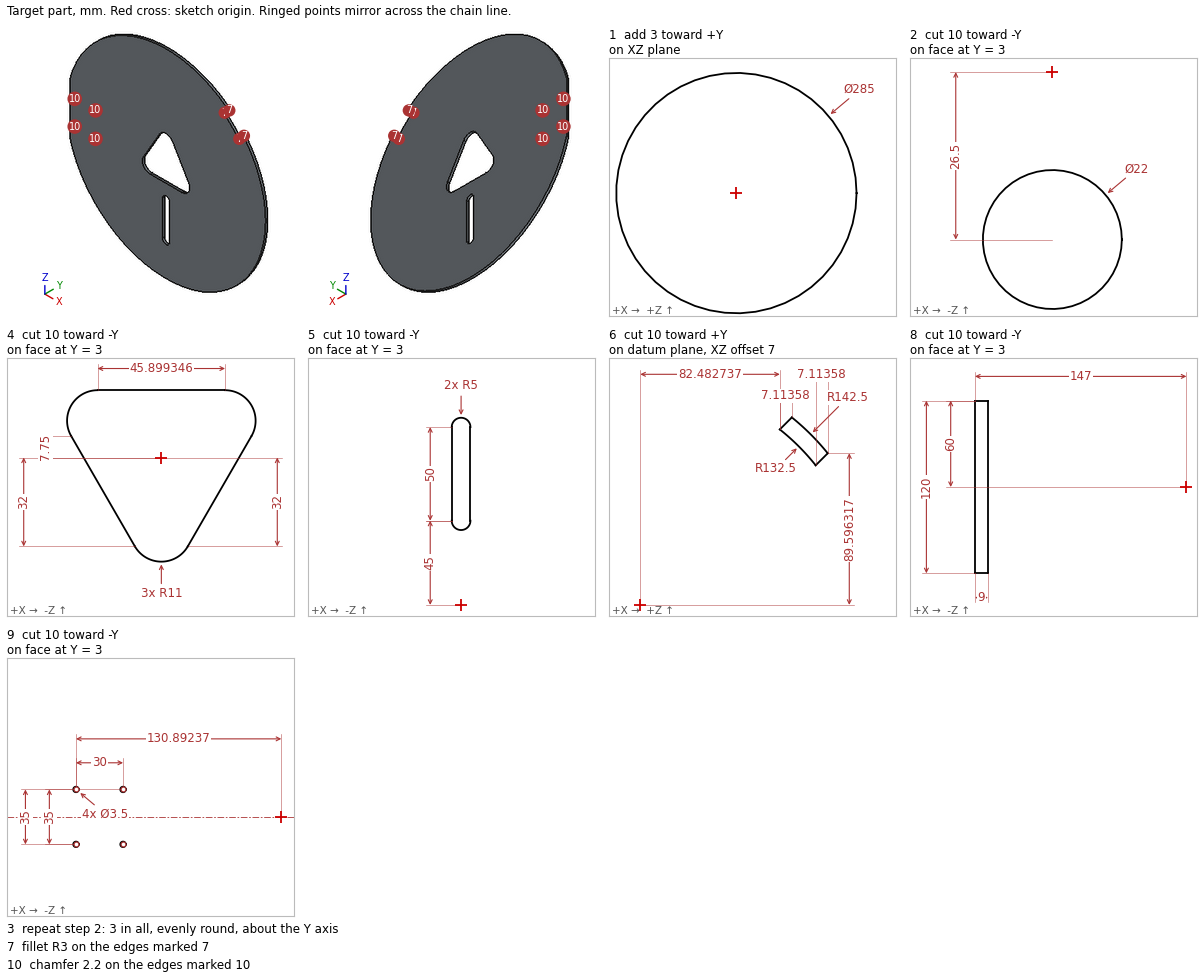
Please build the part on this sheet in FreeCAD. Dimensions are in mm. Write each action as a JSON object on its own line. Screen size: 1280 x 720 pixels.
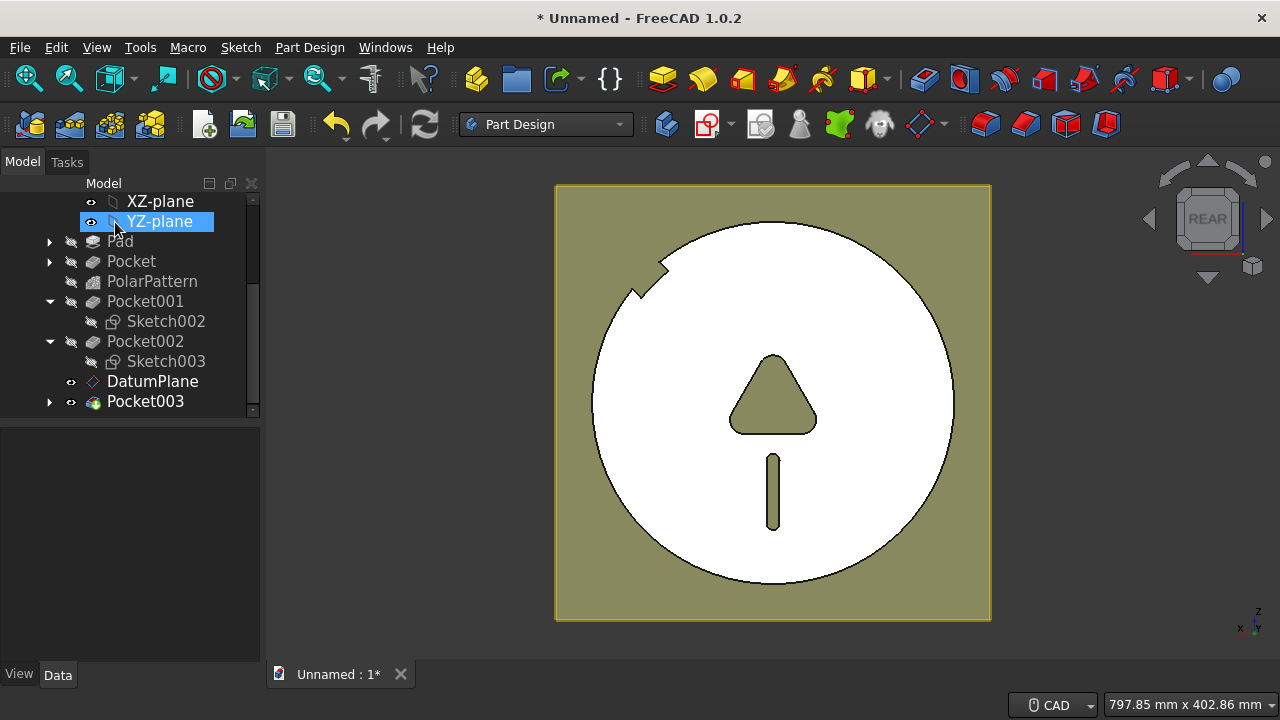
{"action": "left_click", "coordinate": [116, 382]}
{"action": "key", "text": "space"}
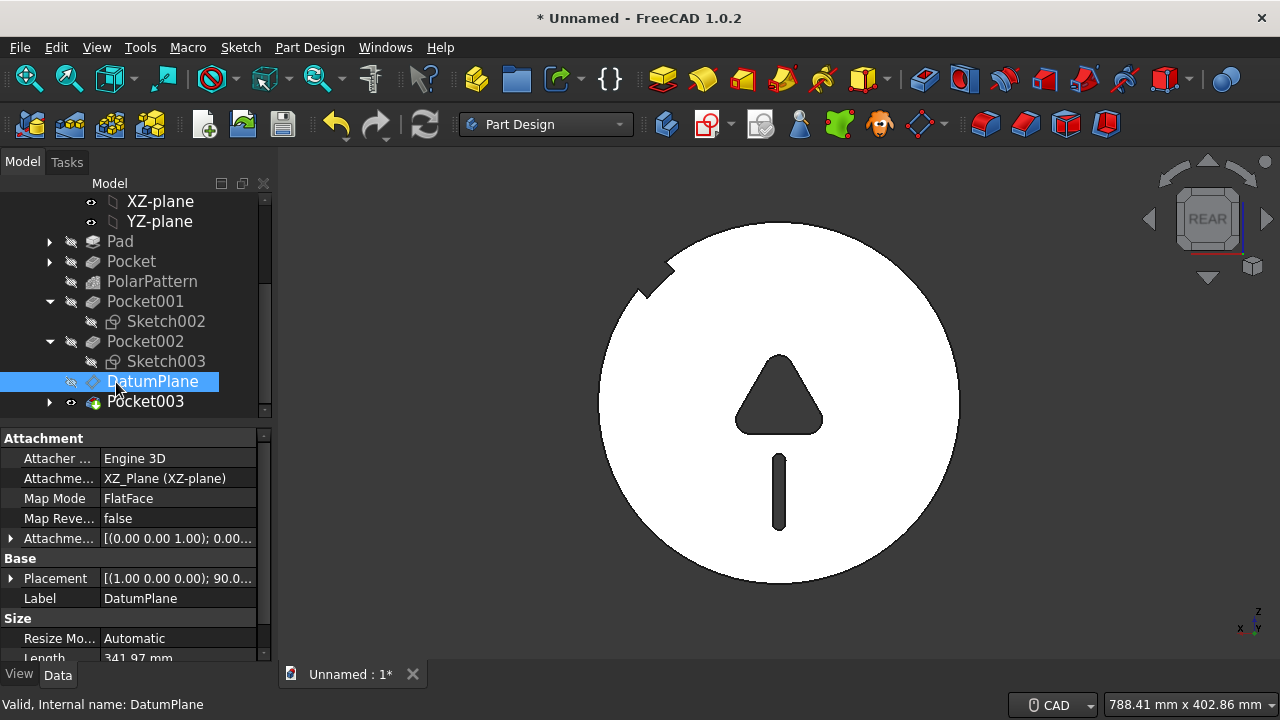
{"action": "scroll", "coordinate": [674, 270], "scroll_direction": "up", "scroll_amount": 12}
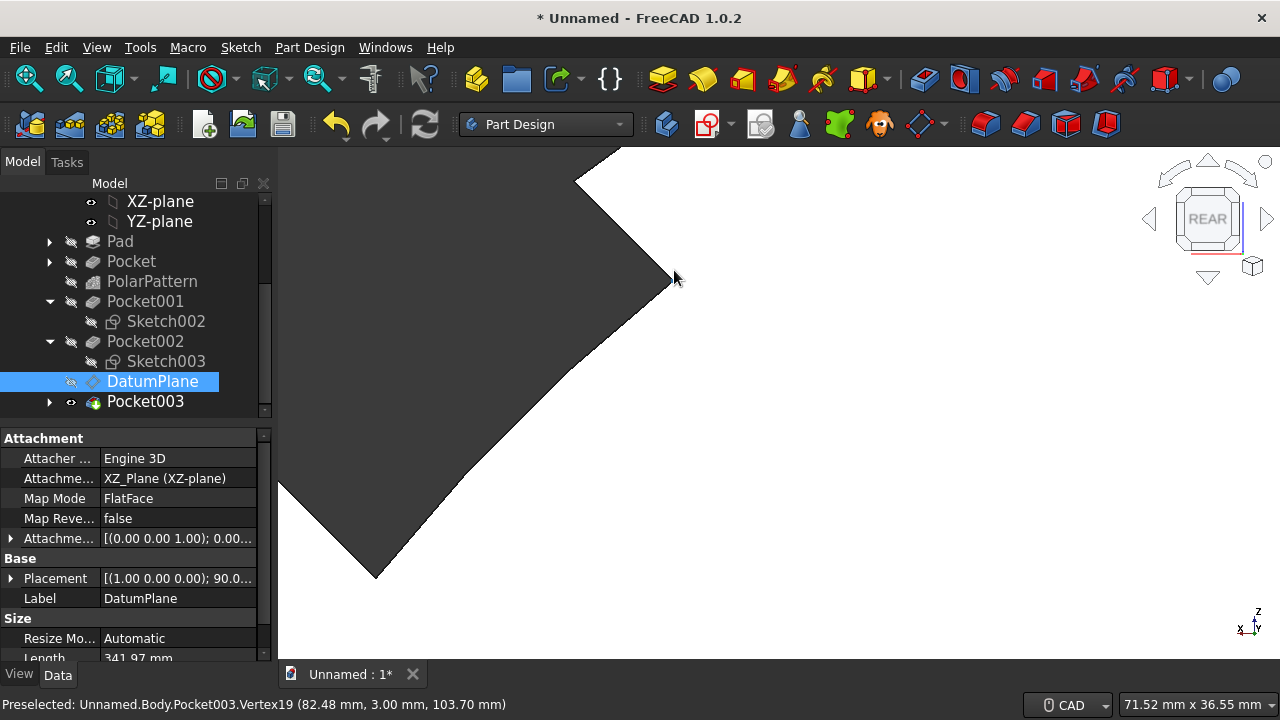
{"action": "key", "text": "v f"}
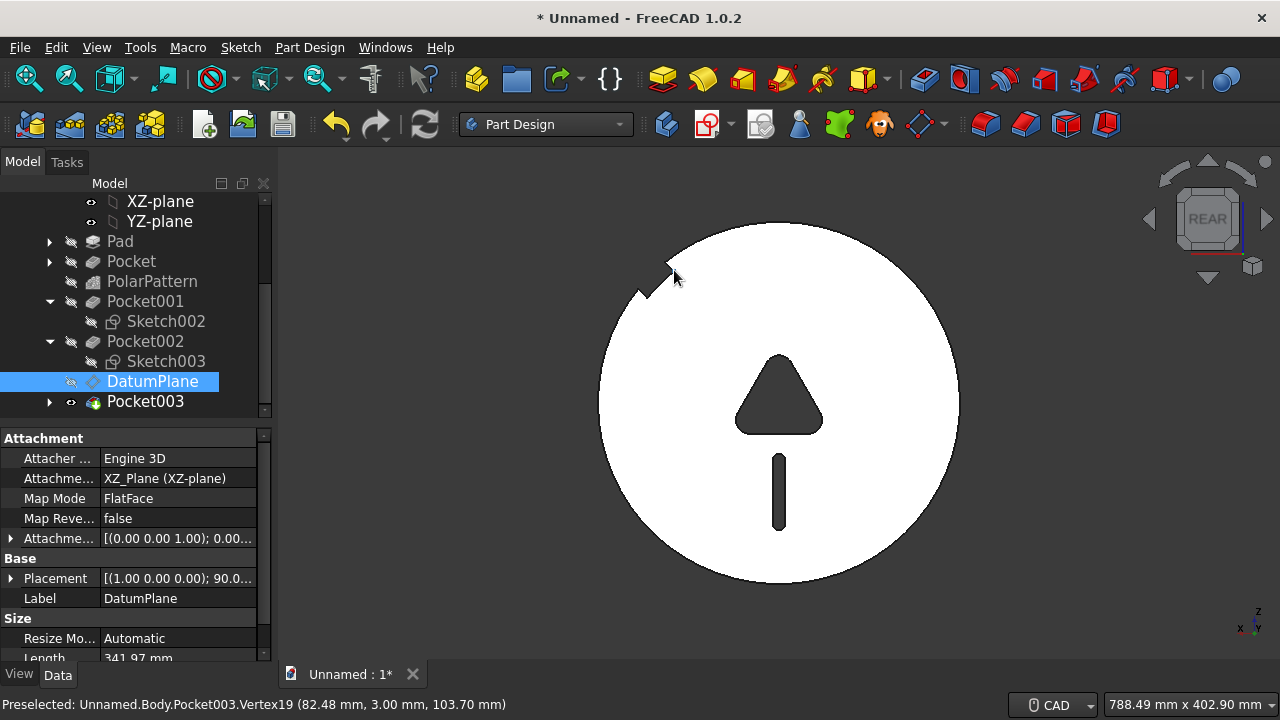
{"action": "key", "text": "0"}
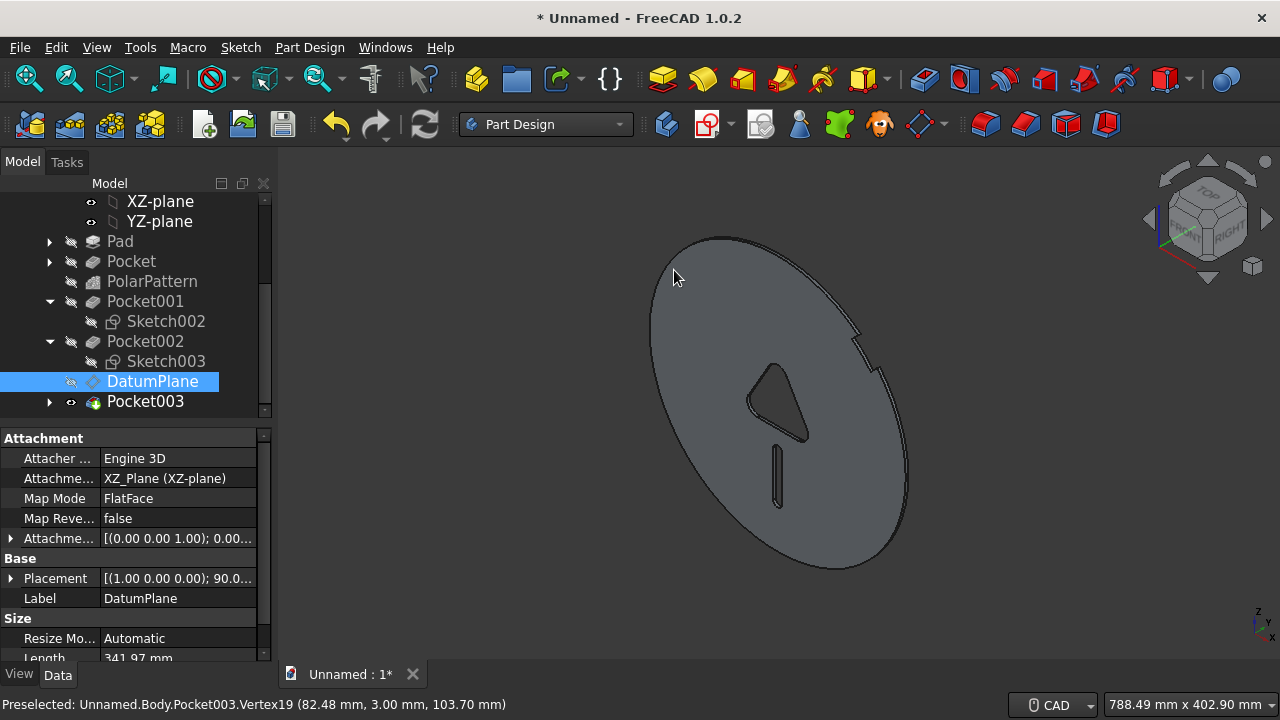
{"action": "scroll", "coordinate": [853, 337], "scroll_direction": "up", "scroll_amount": 12}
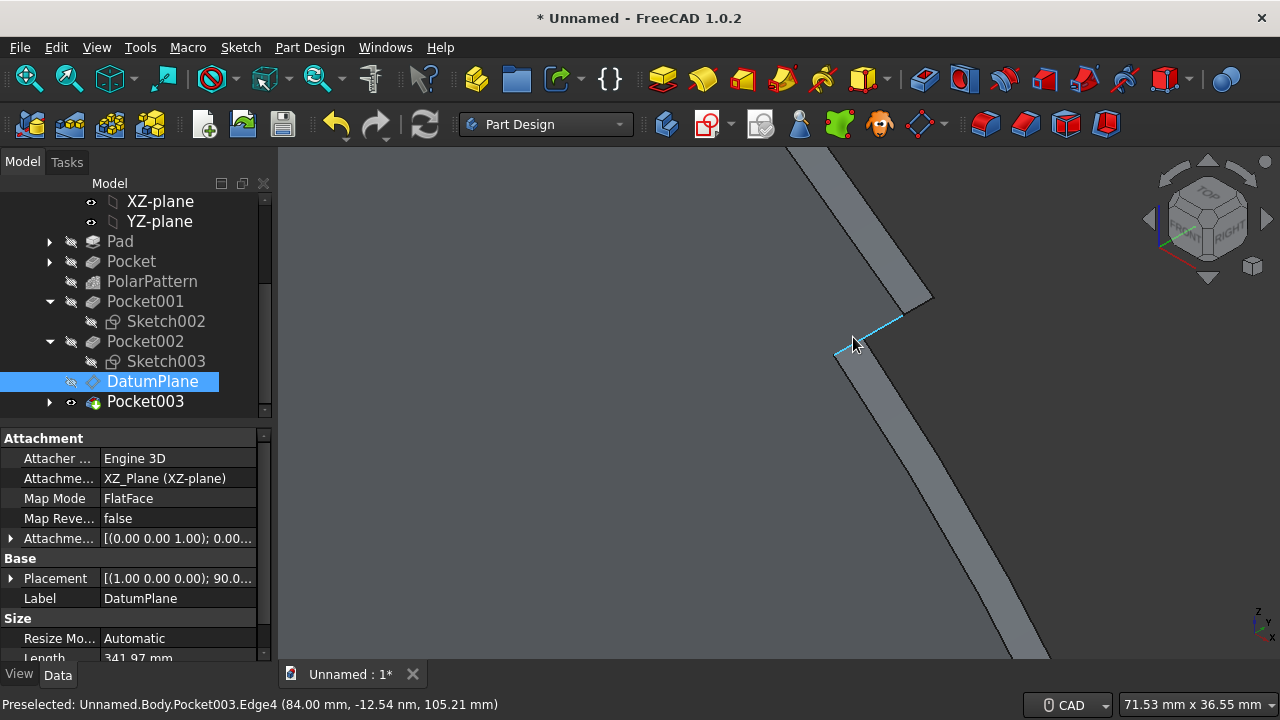
{"action": "left_click", "coordinate": [919, 305]}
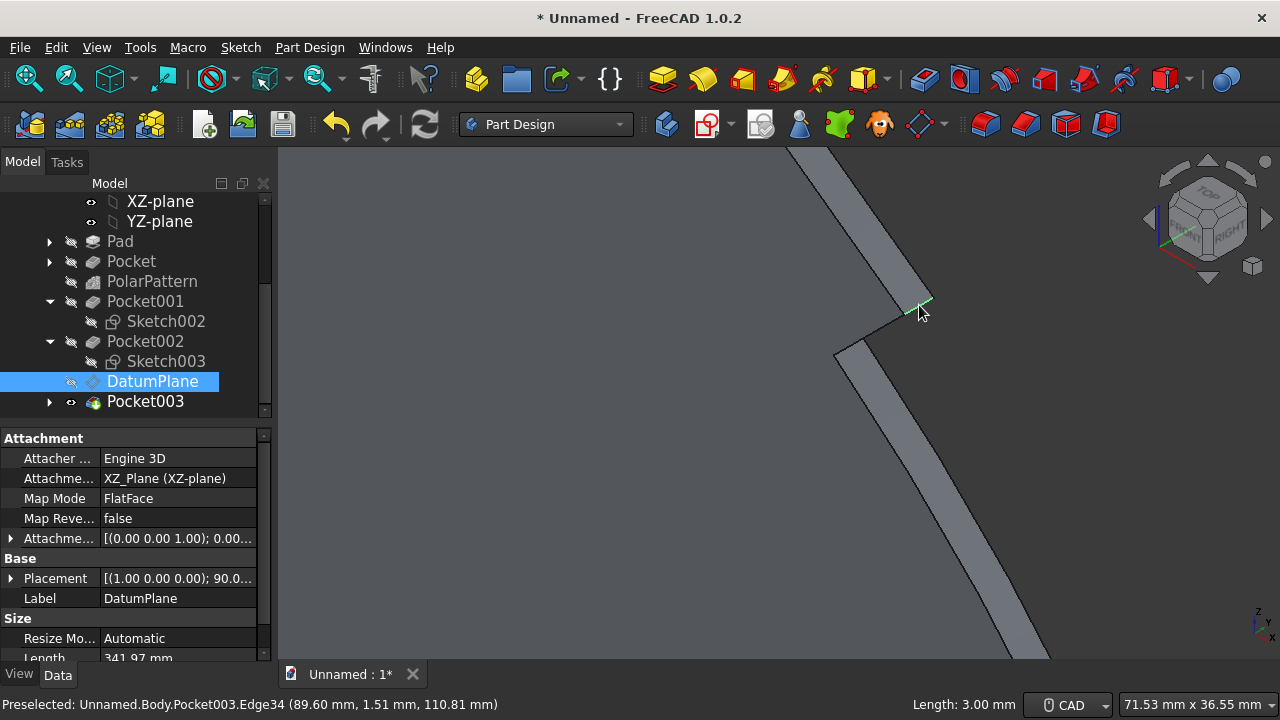
{"action": "left_click", "coordinate": [30, 80]}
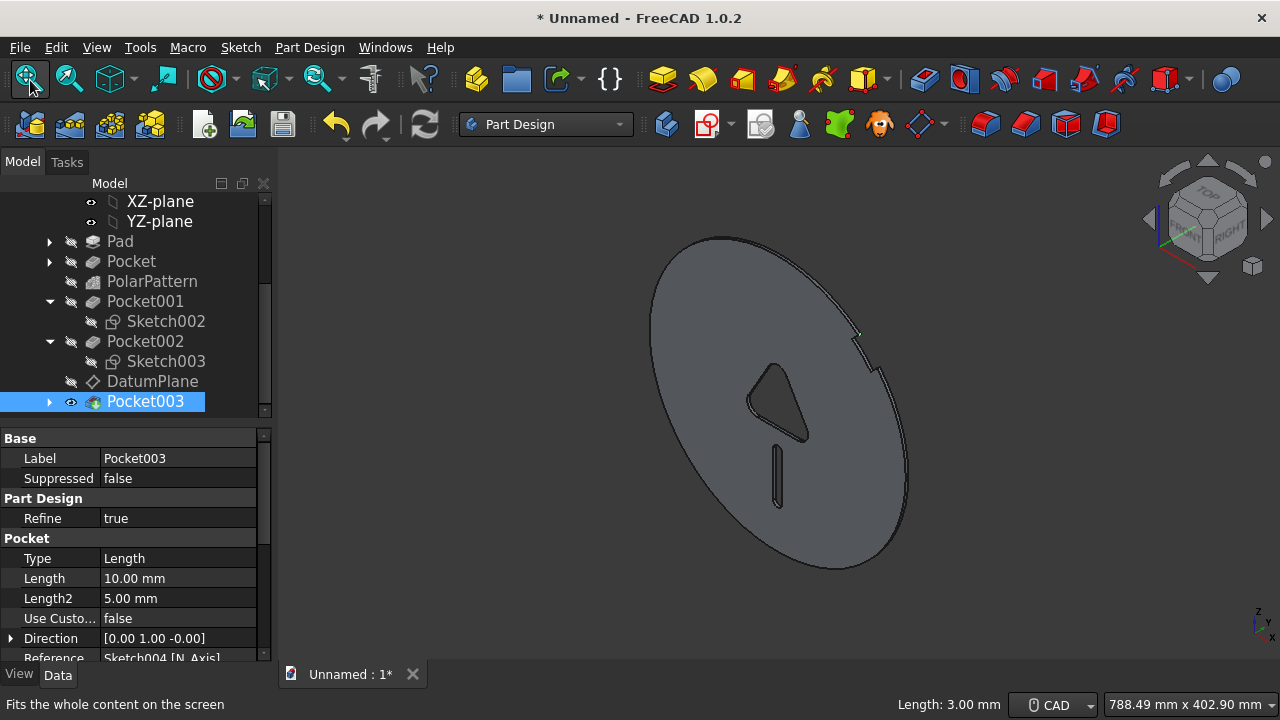
{"action": "key", "text": "2"}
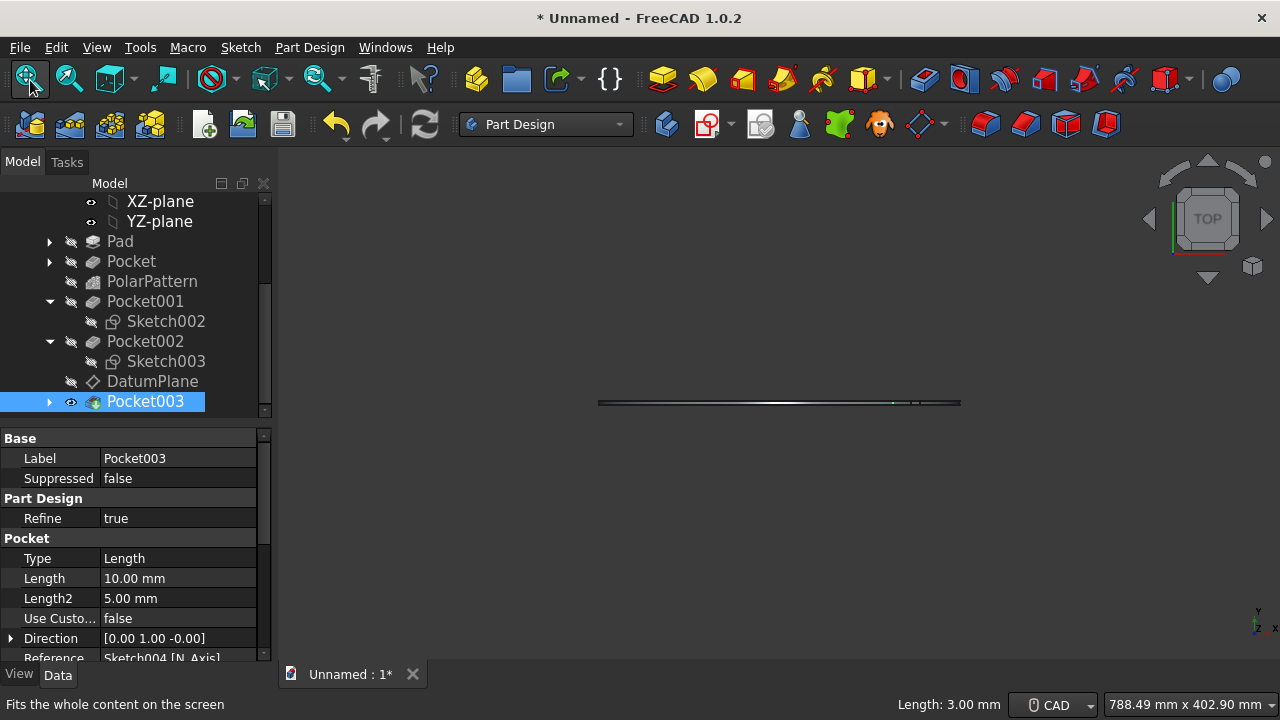
{"action": "left_click", "coordinate": [30, 80]}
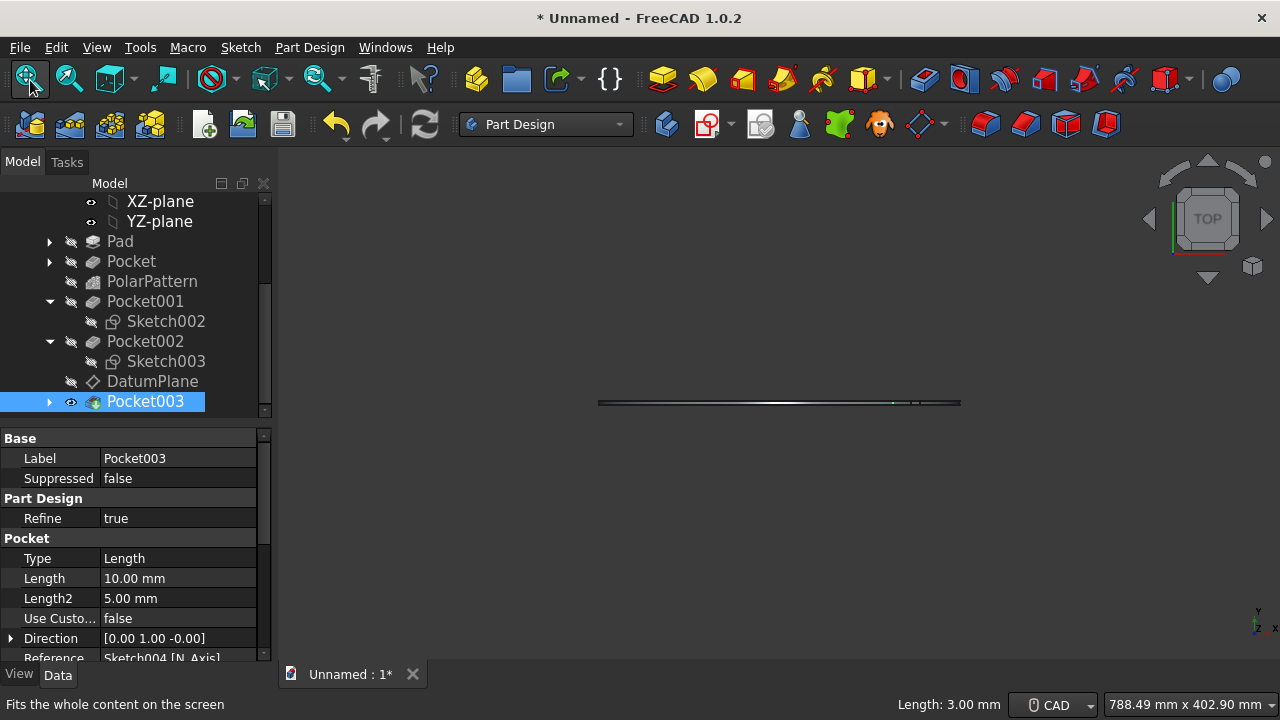
{"action": "scroll", "coordinate": [884, 402], "scroll_direction": "up", "scroll_amount": 12}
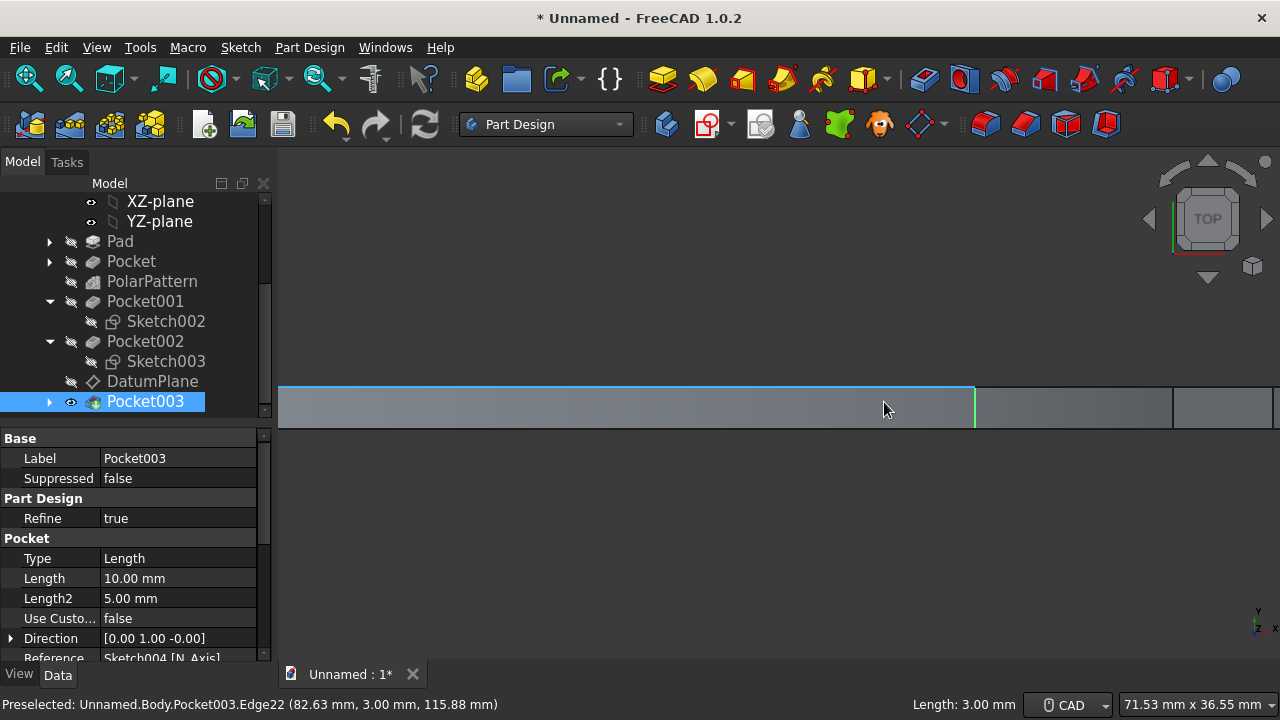
{"action": "left_click", "coordinate": [30, 80]}